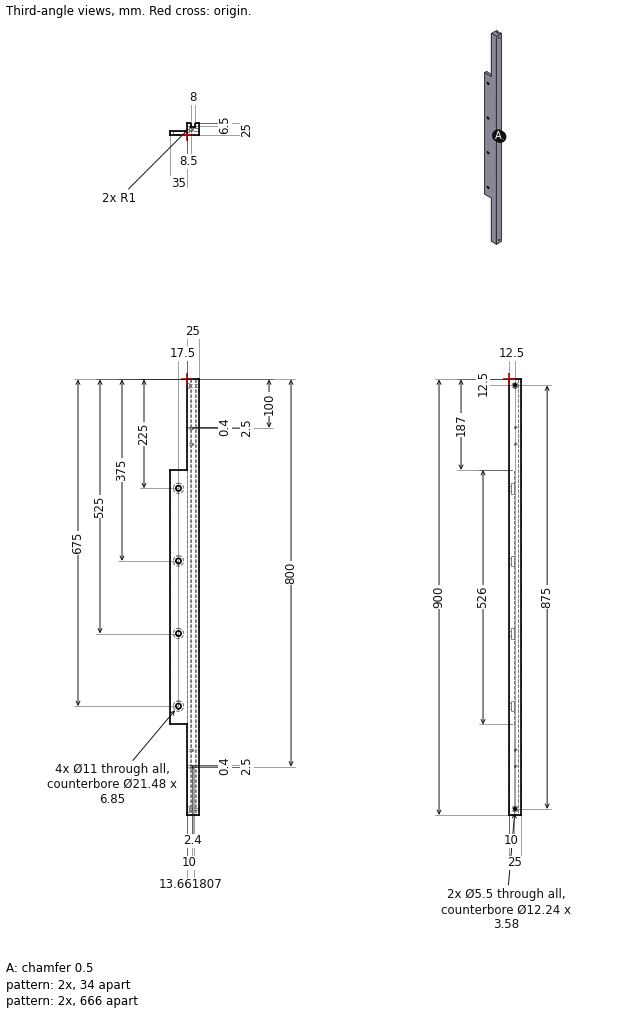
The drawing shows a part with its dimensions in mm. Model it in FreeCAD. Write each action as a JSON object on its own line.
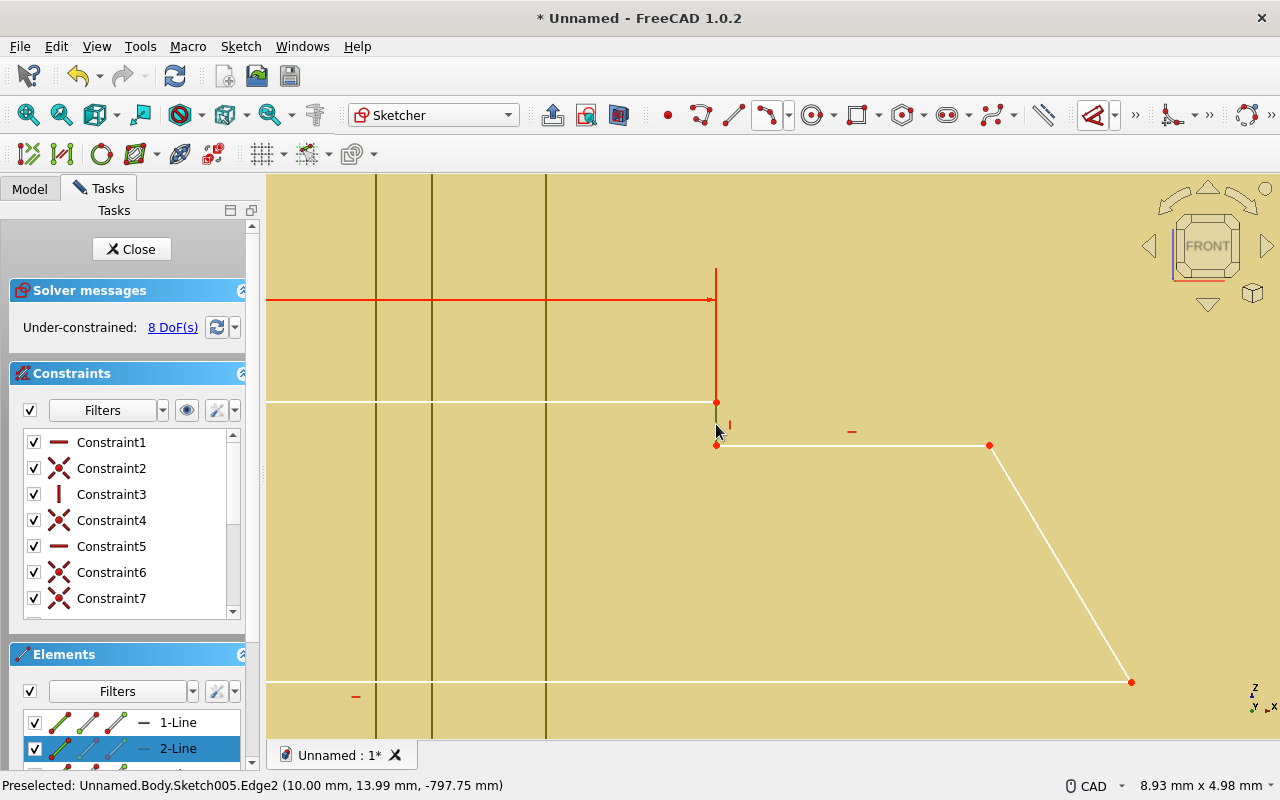
{"action": "key", "text": "i"}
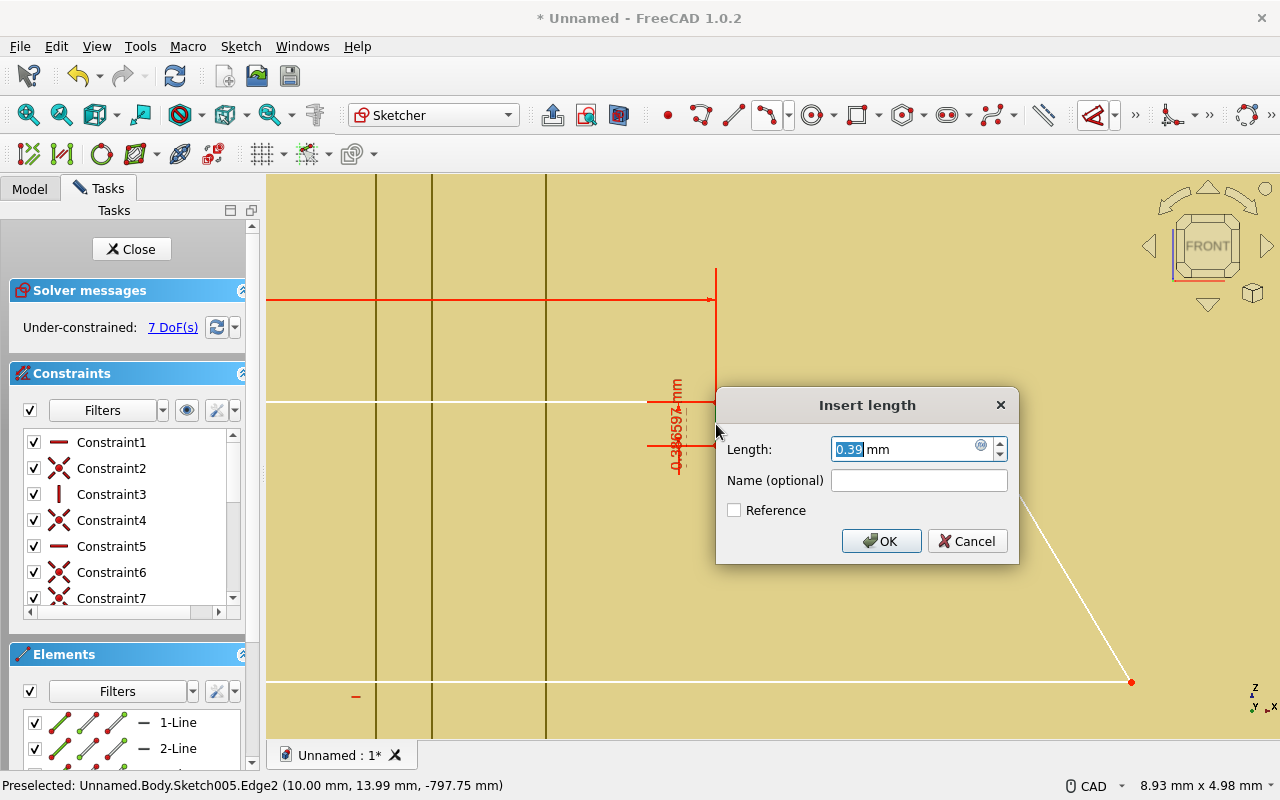
{"action": "type", "text": "0.4"}
{"action": "key", "text": "Return"}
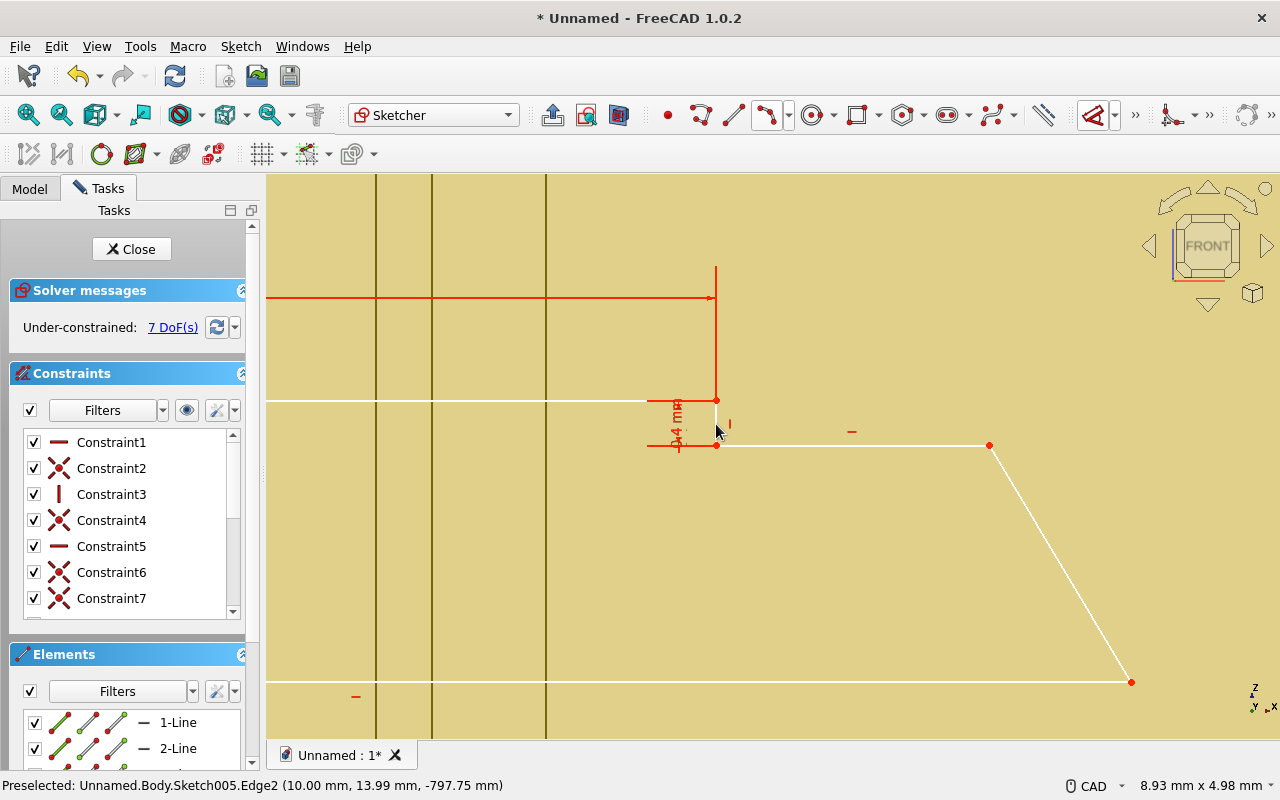
{"action": "scroll", "coordinate": [717, 430], "scroll_direction": "down", "scroll_amount": 7}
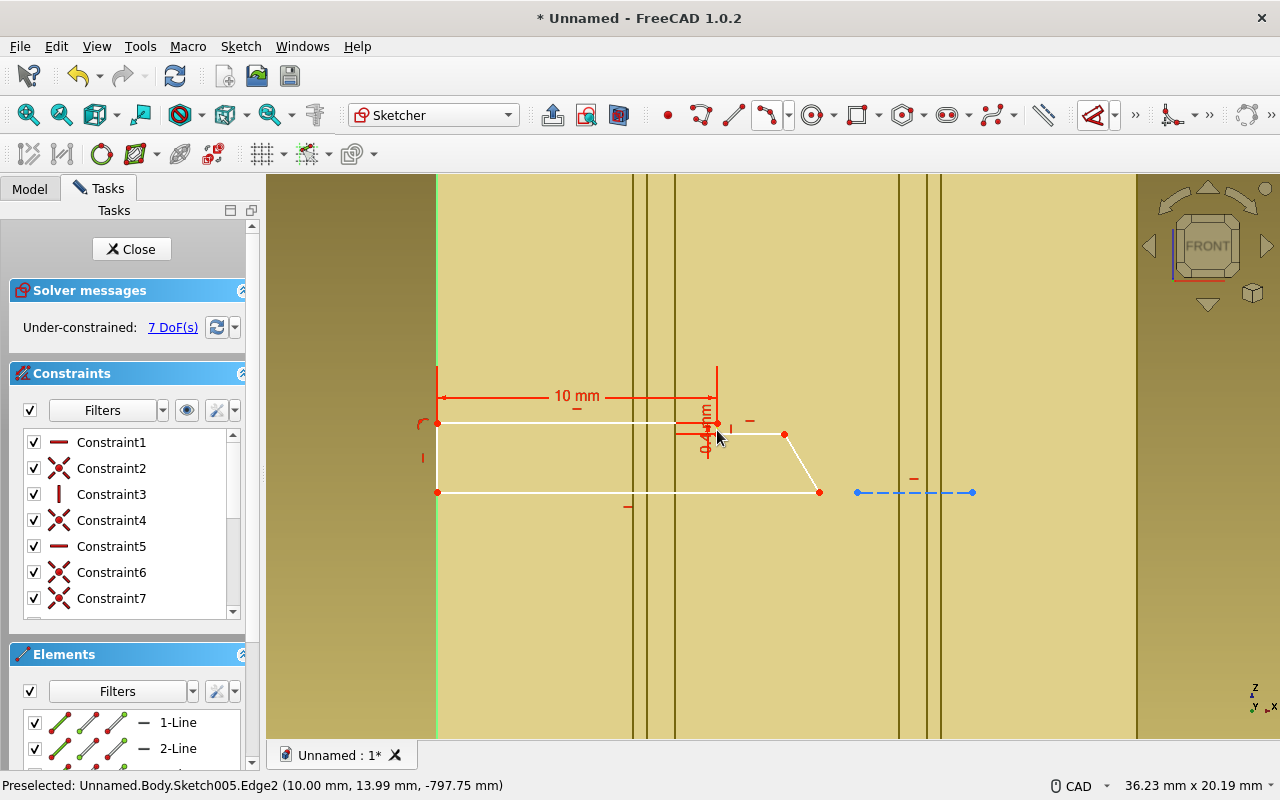
{"action": "left_click", "coordinate": [737, 434]}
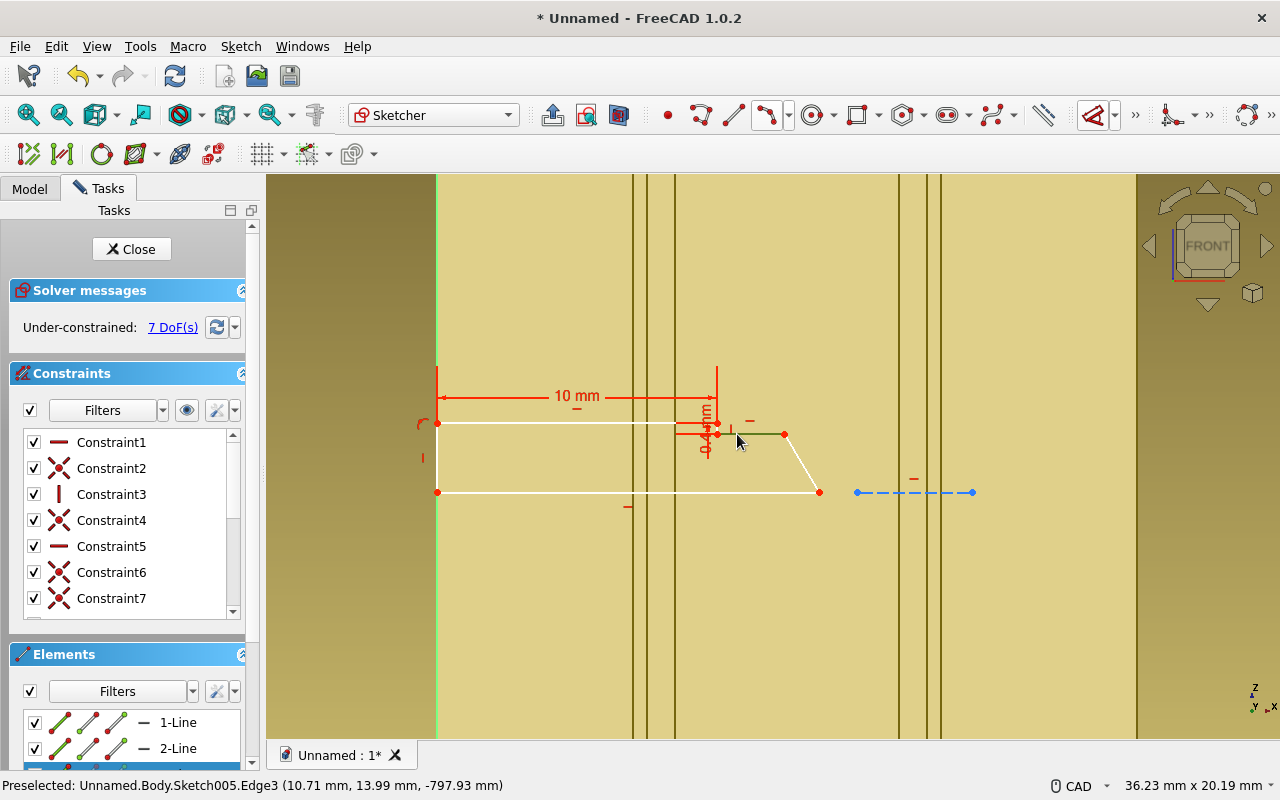
{"action": "left_click", "coordinate": [1114, 116]}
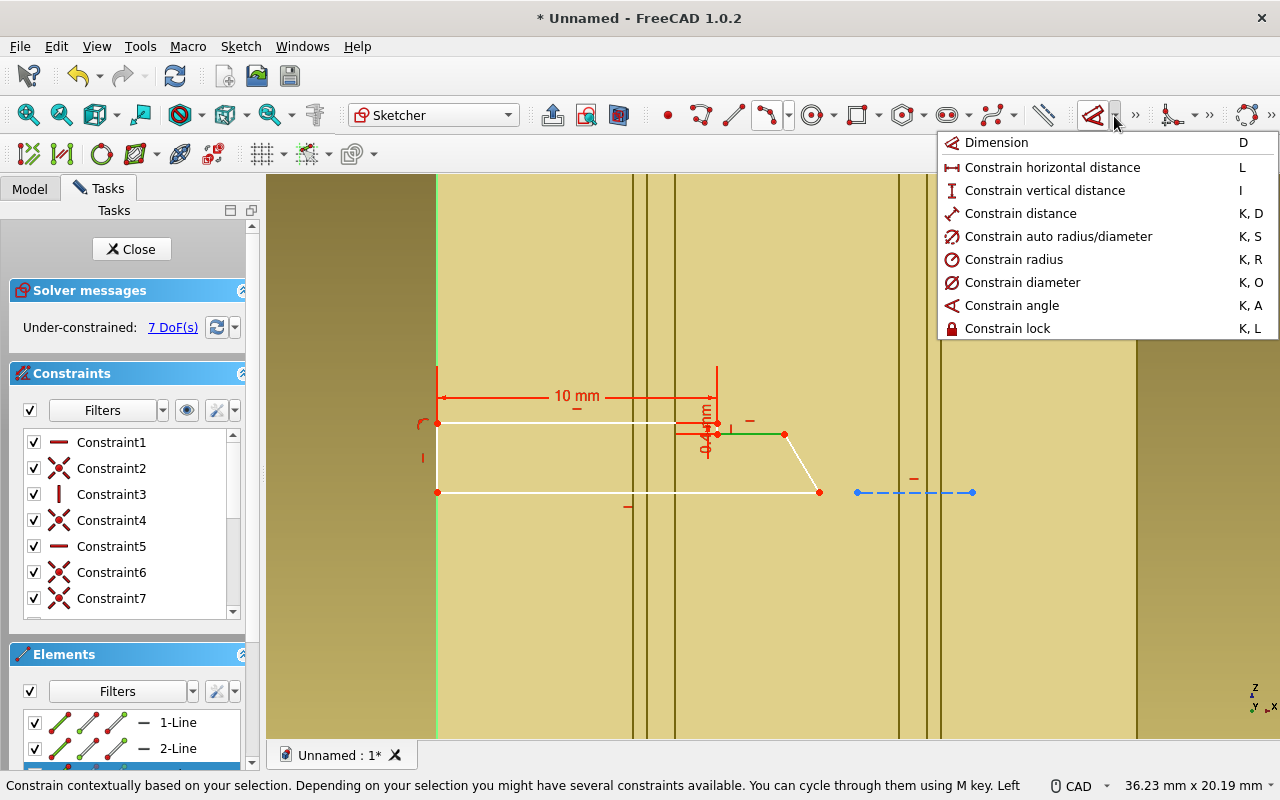
{"action": "left_click", "coordinate": [1108, 168]}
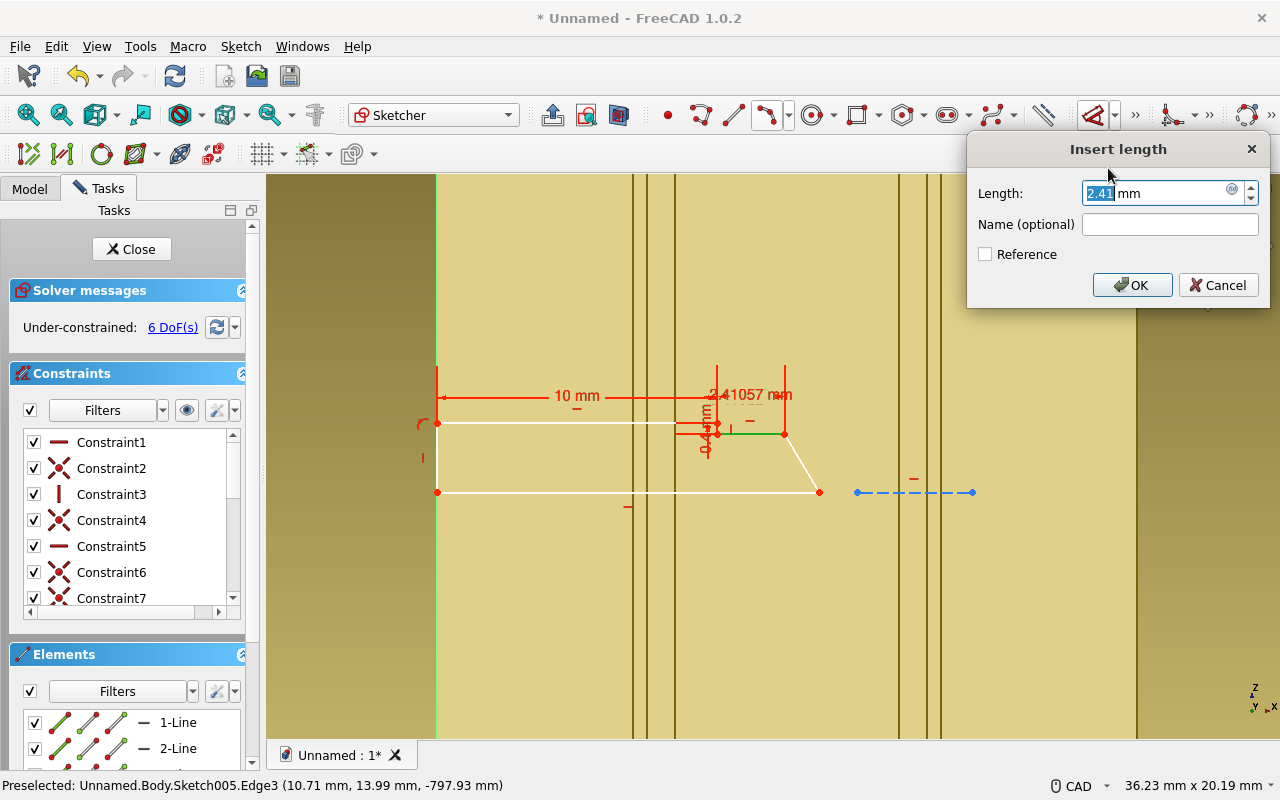
{"action": "type", "text": "2.4"}
{"action": "key", "text": "Return"}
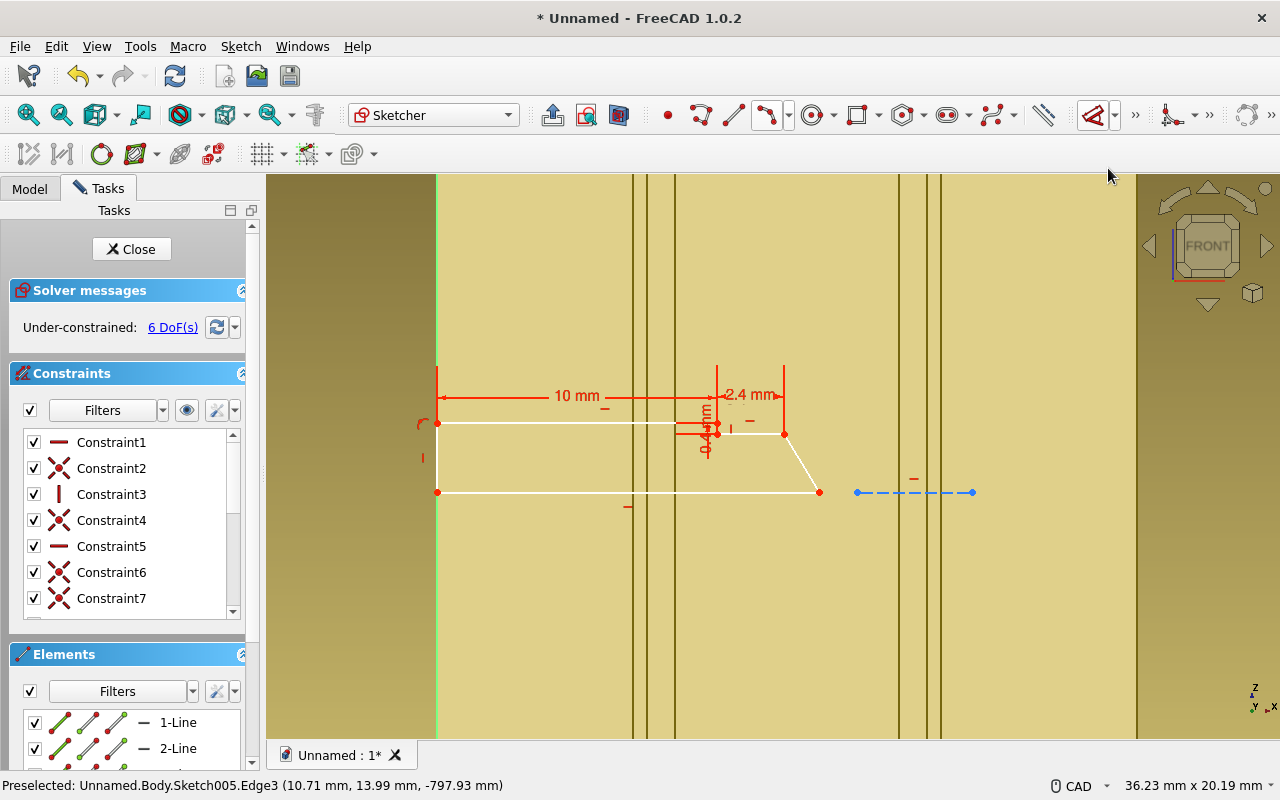
{"action": "left_click", "coordinate": [437, 472]}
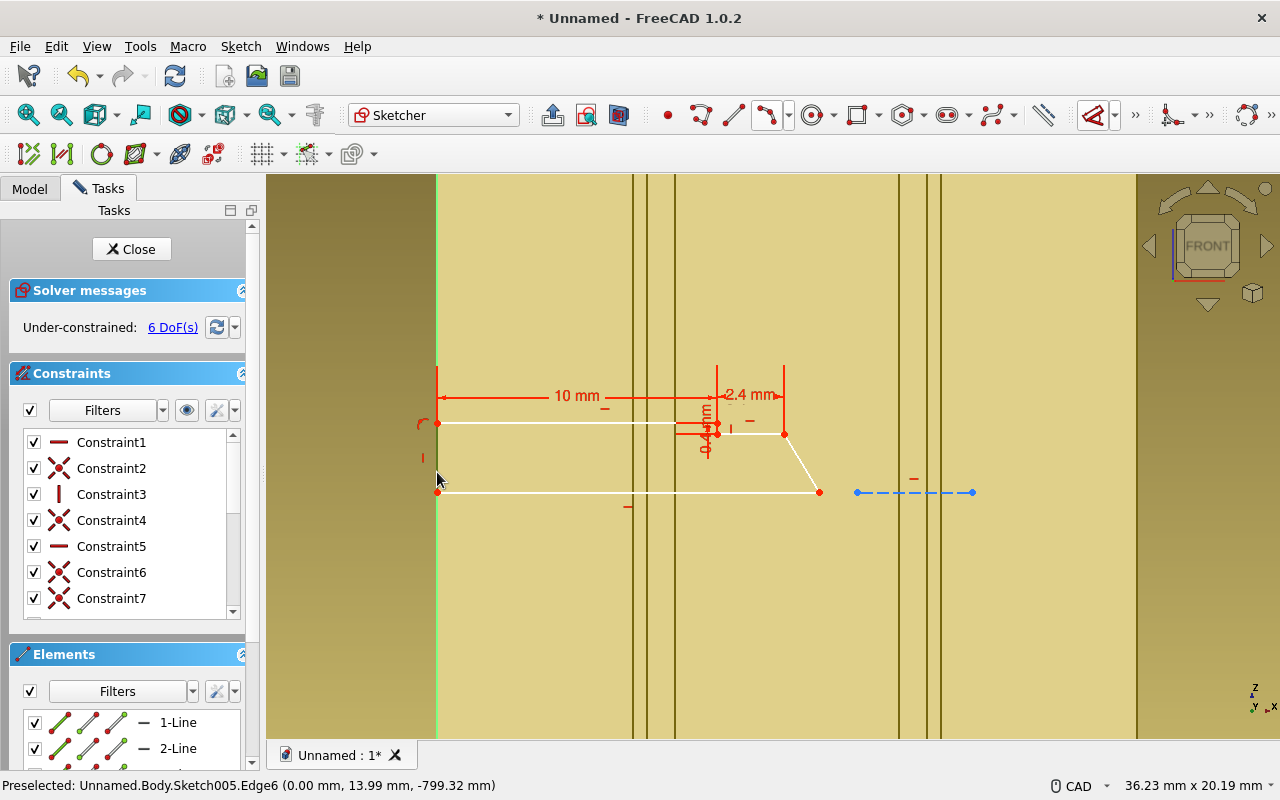
{"action": "left_click", "coordinate": [1114, 116]}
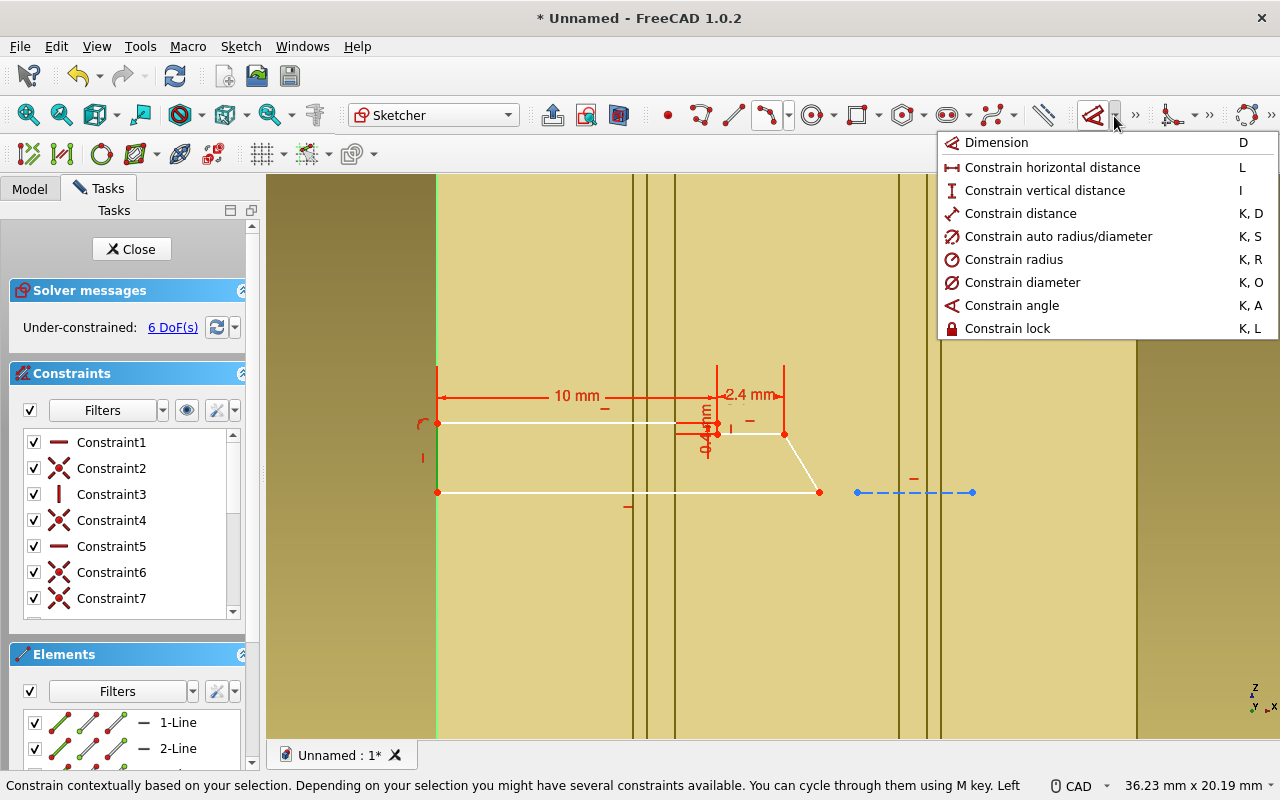
{"action": "left_click", "coordinate": [1108, 190]}